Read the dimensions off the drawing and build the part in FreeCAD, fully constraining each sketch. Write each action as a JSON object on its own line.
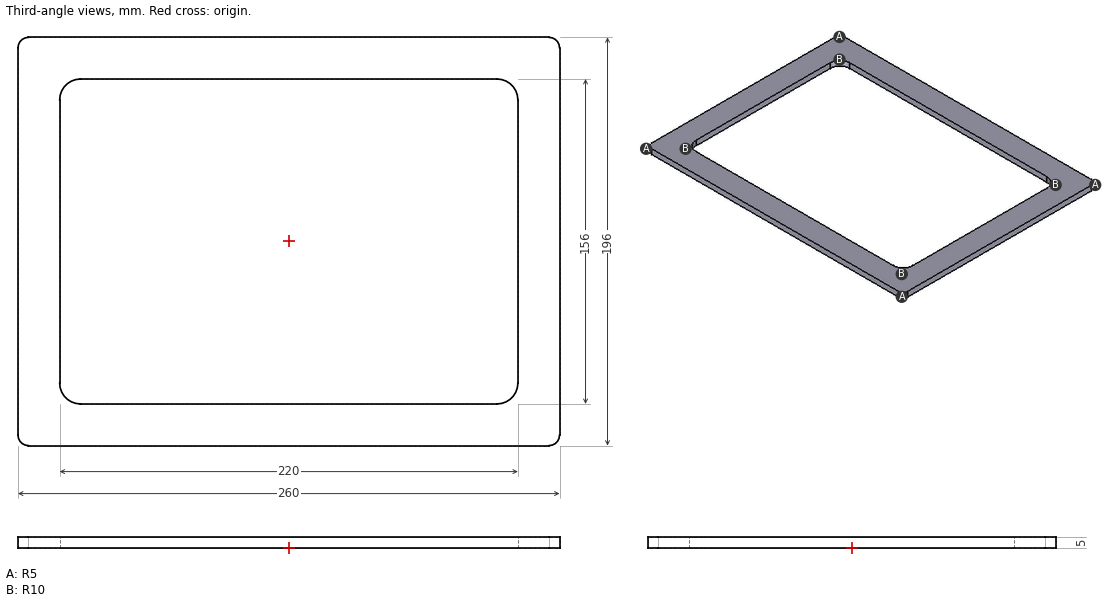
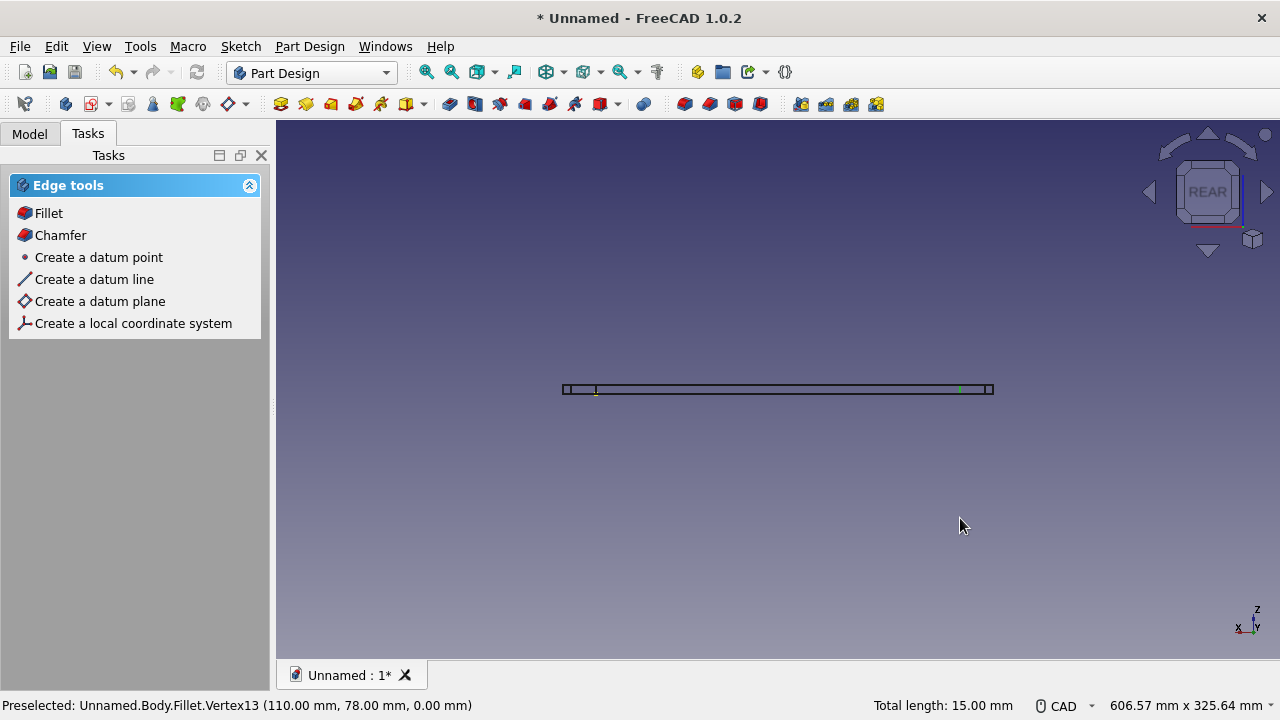
{"action": "key", "text": "v f"}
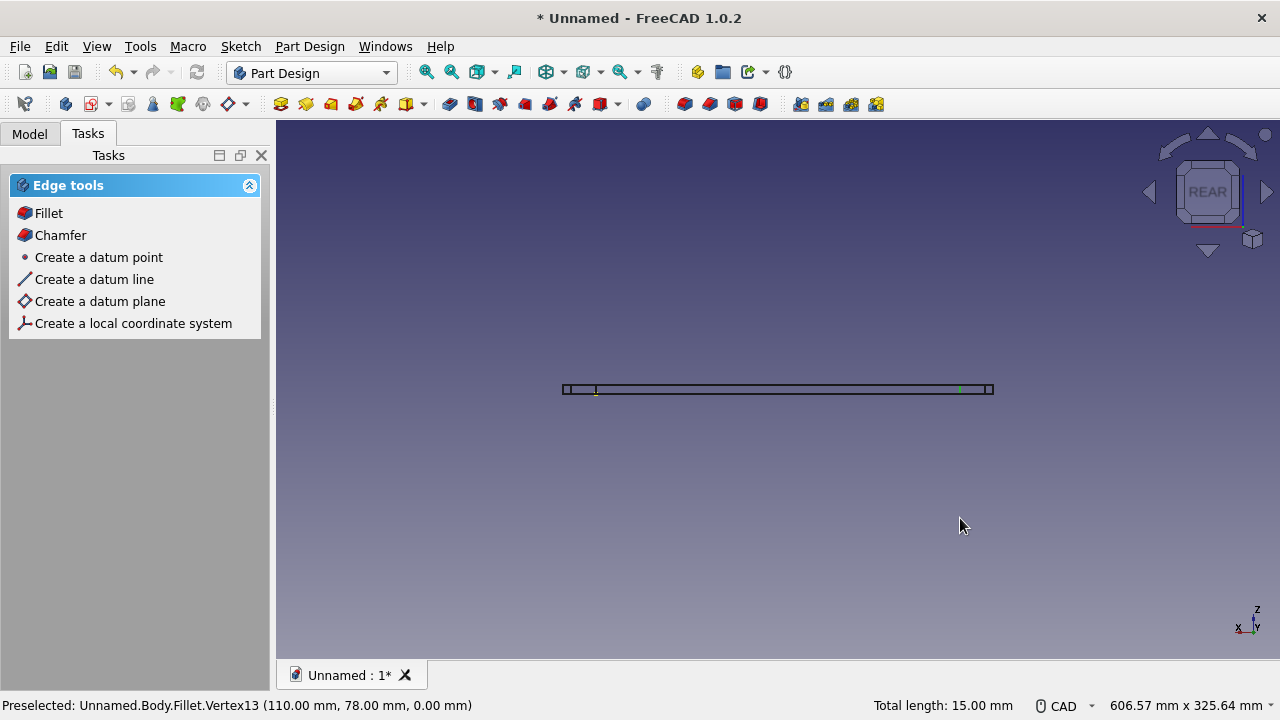
{"action": "scroll", "coordinate": [596, 389], "scroll_direction": "up", "scroll_amount": 8}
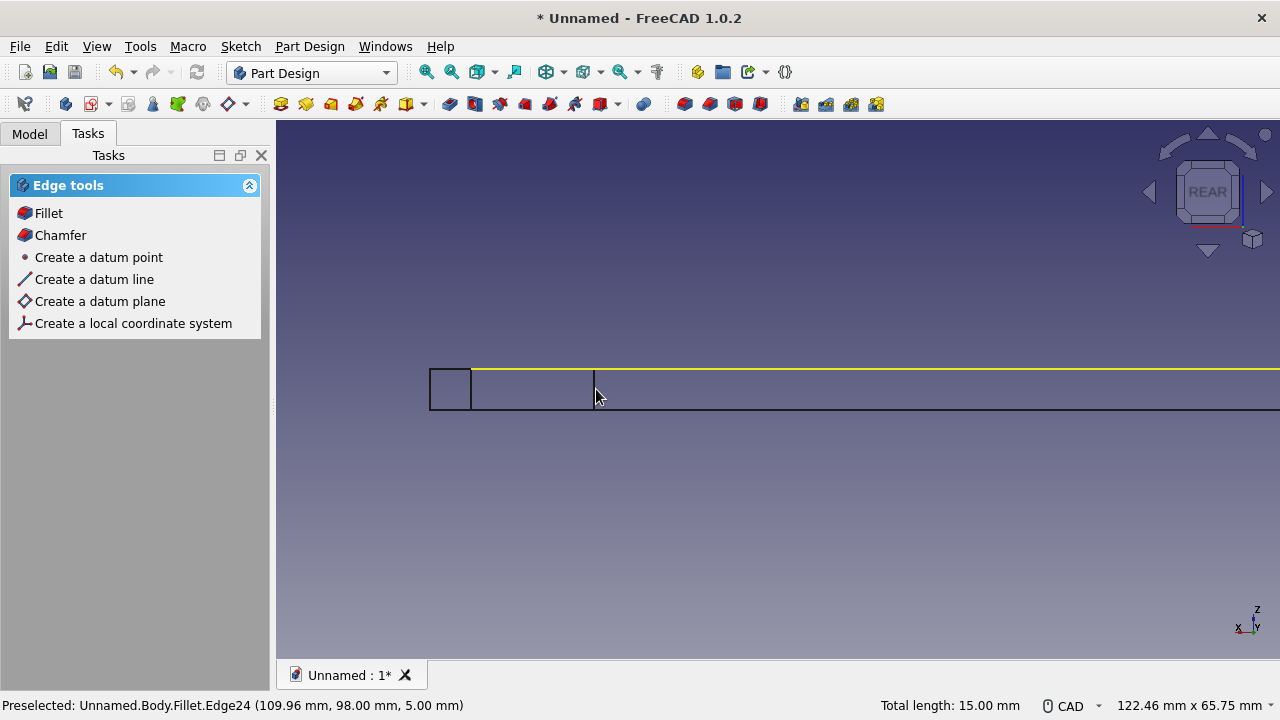
{"action": "left_click", "coordinate": [594, 389], "text": "ctrl"}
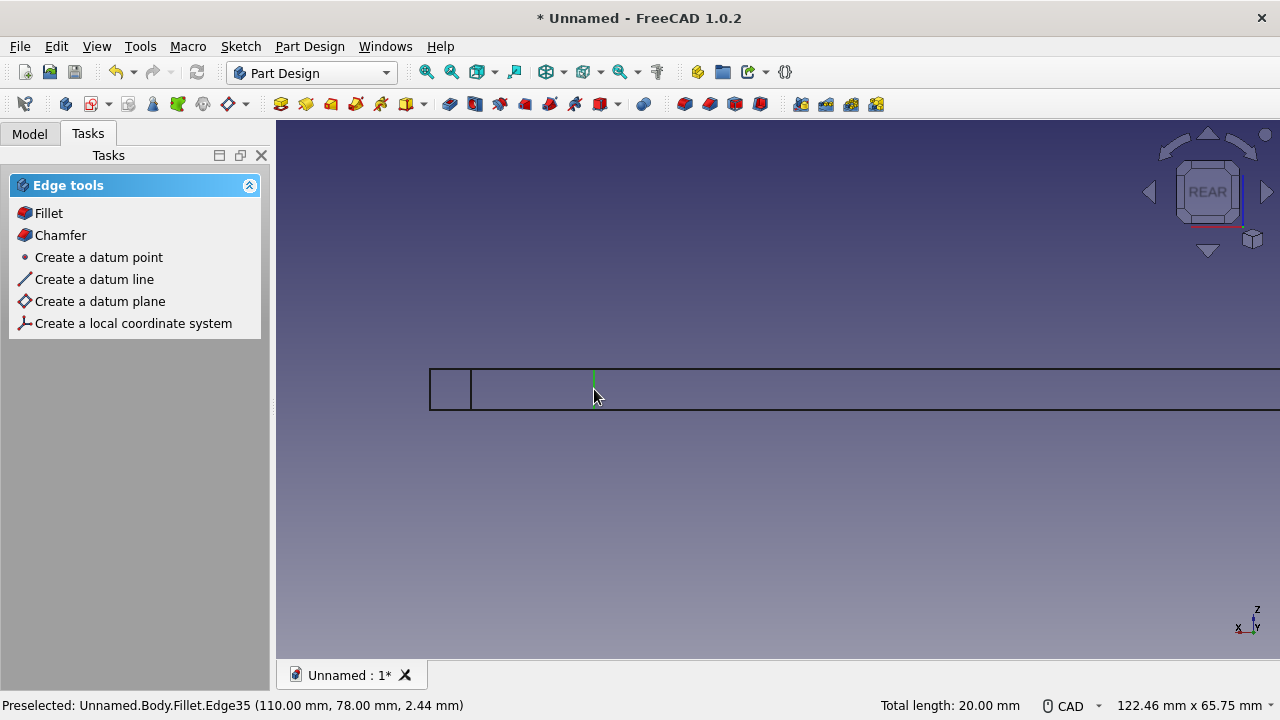
{"action": "key", "text": "v 1"}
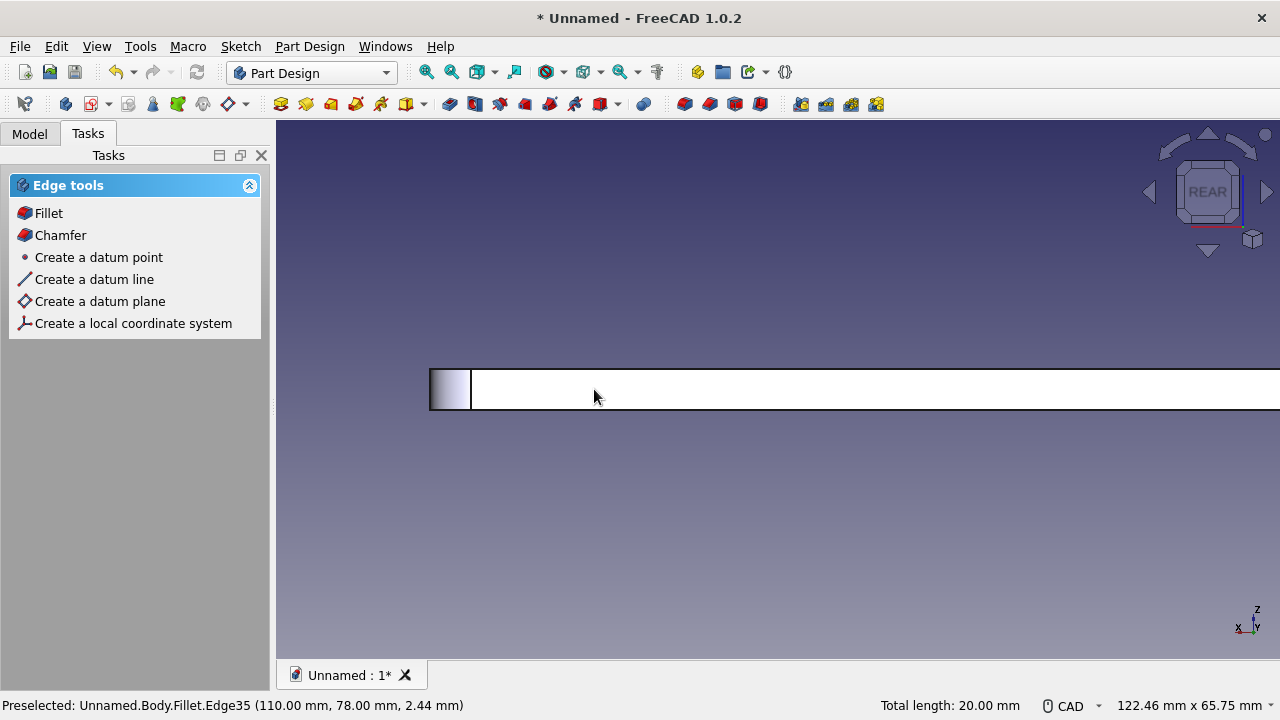
{"action": "left_click", "coordinate": [685, 104]}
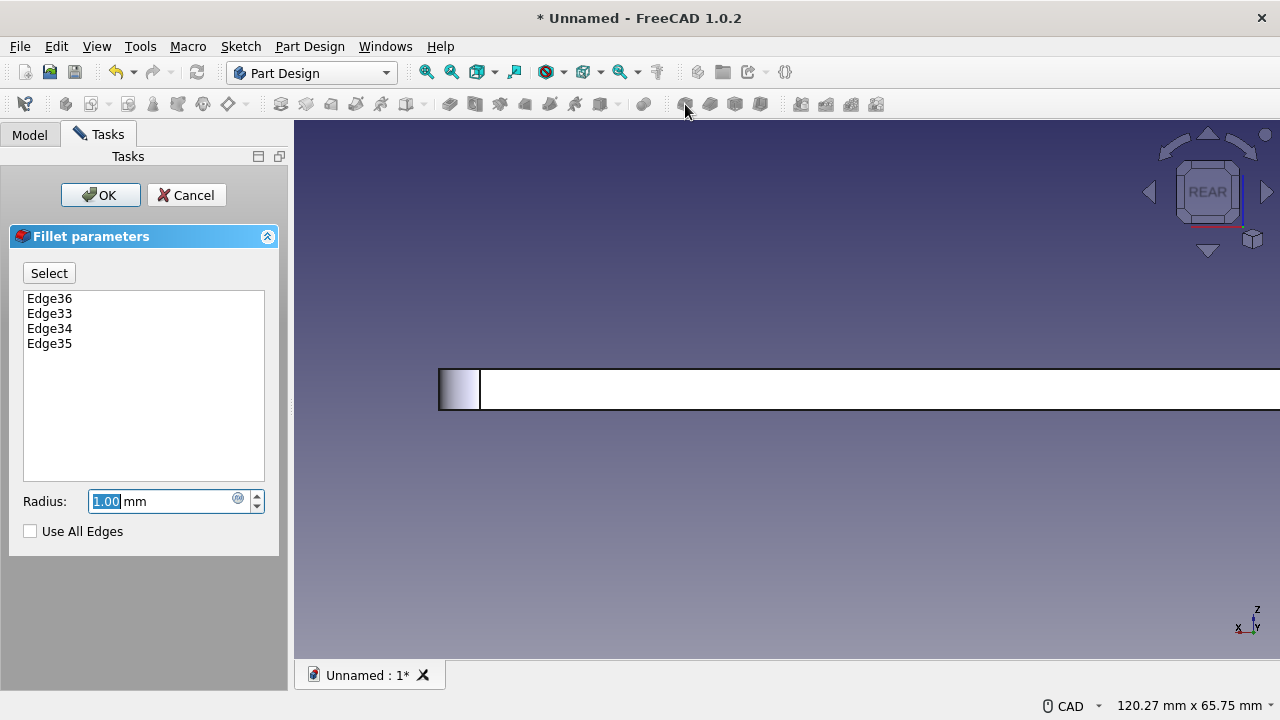
{"action": "type", "text": "10"}
{"action": "key", "text": "Tab"}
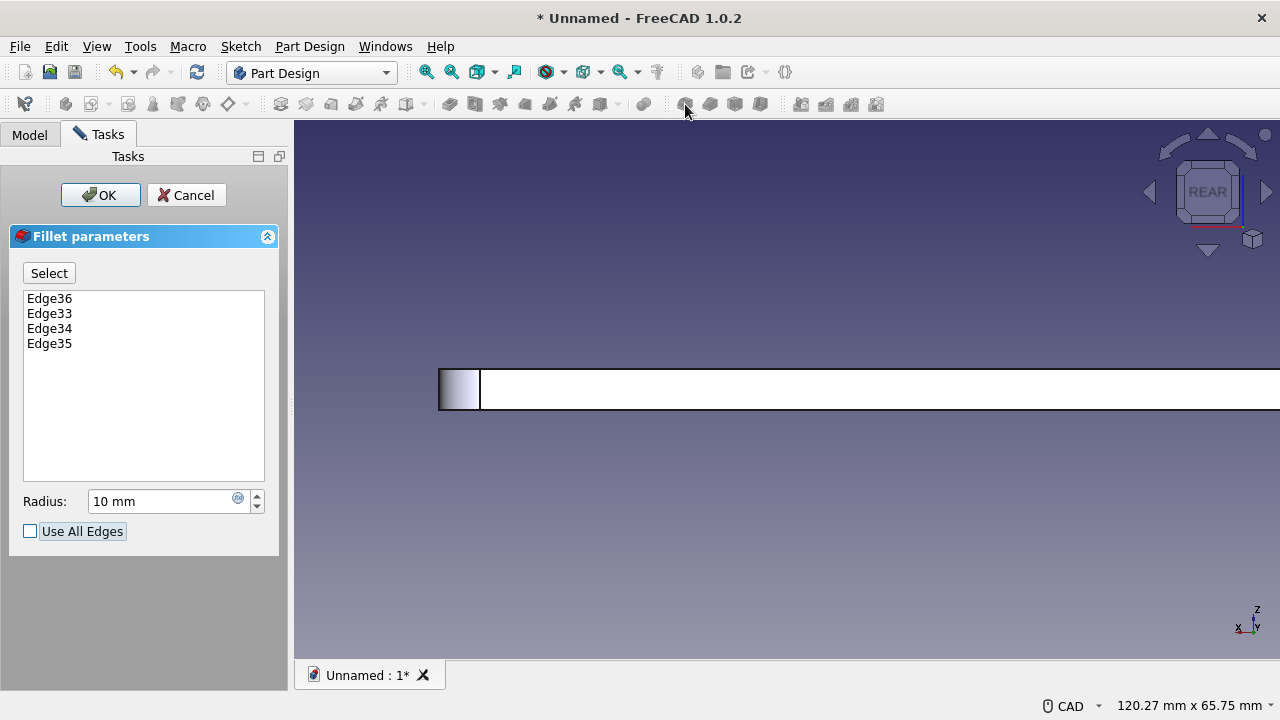
{"action": "left_click", "coordinate": [101, 195]}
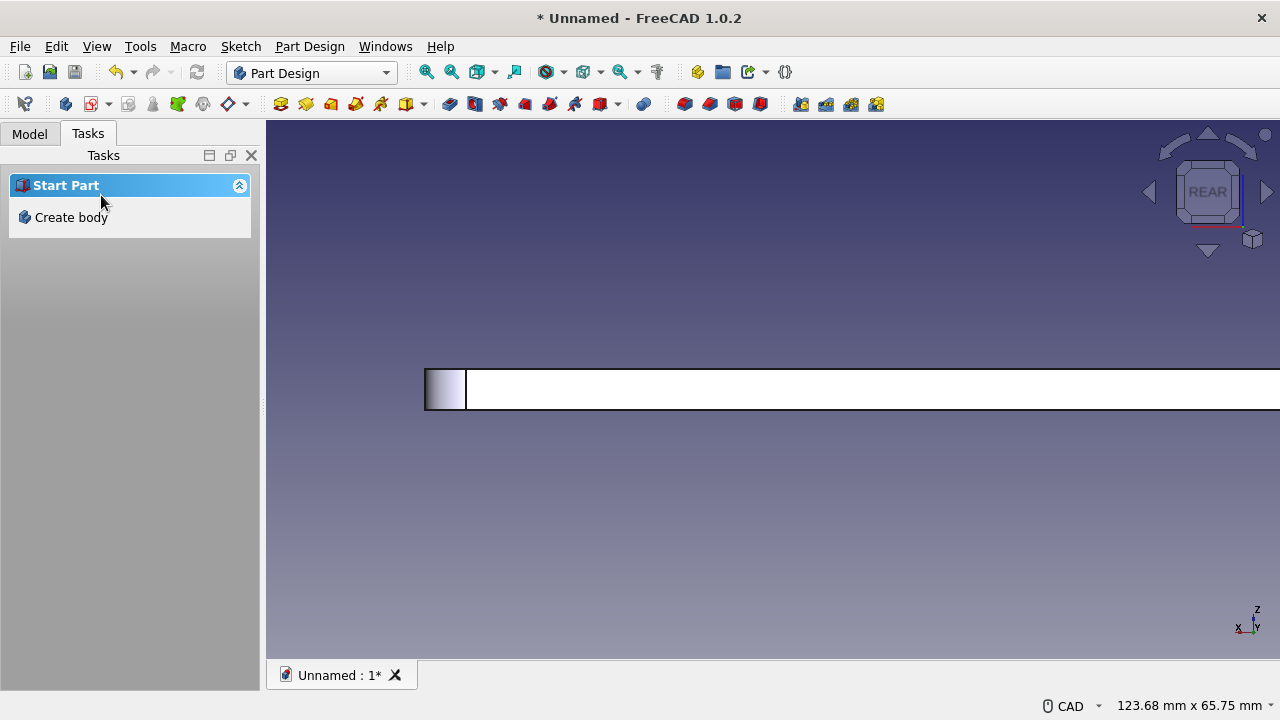
{"action": "key", "text": "0"}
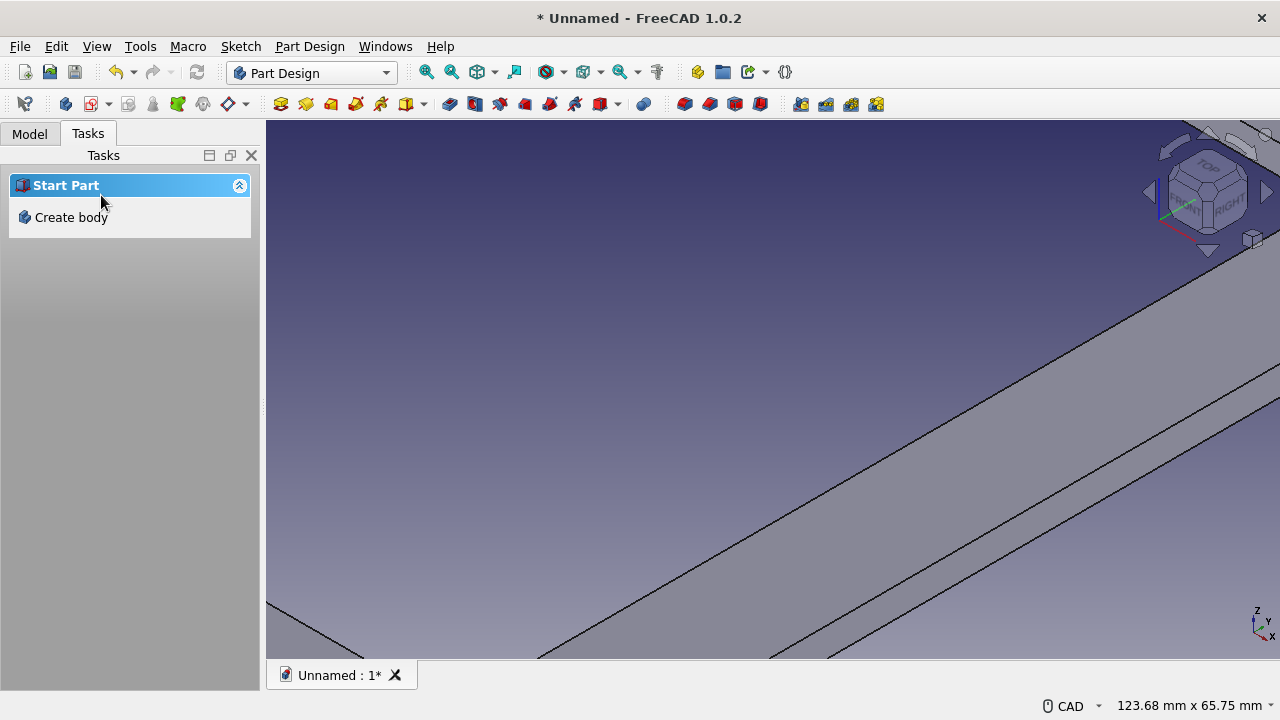
{"action": "left_click", "coordinate": [427, 72]}